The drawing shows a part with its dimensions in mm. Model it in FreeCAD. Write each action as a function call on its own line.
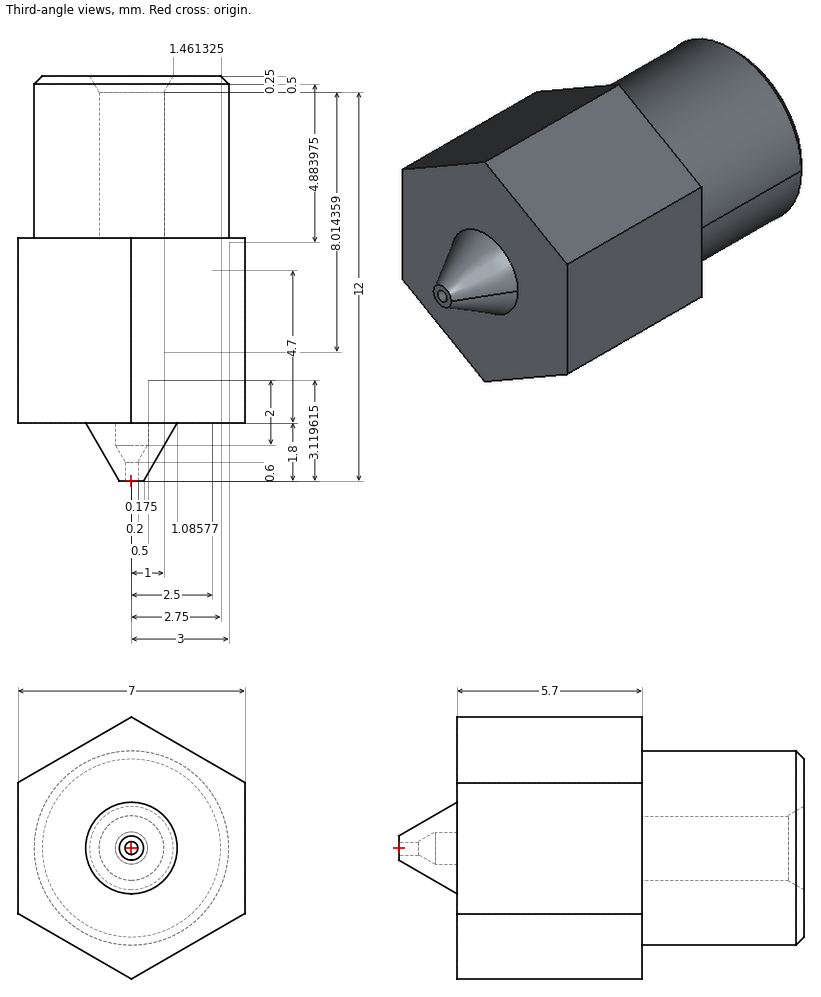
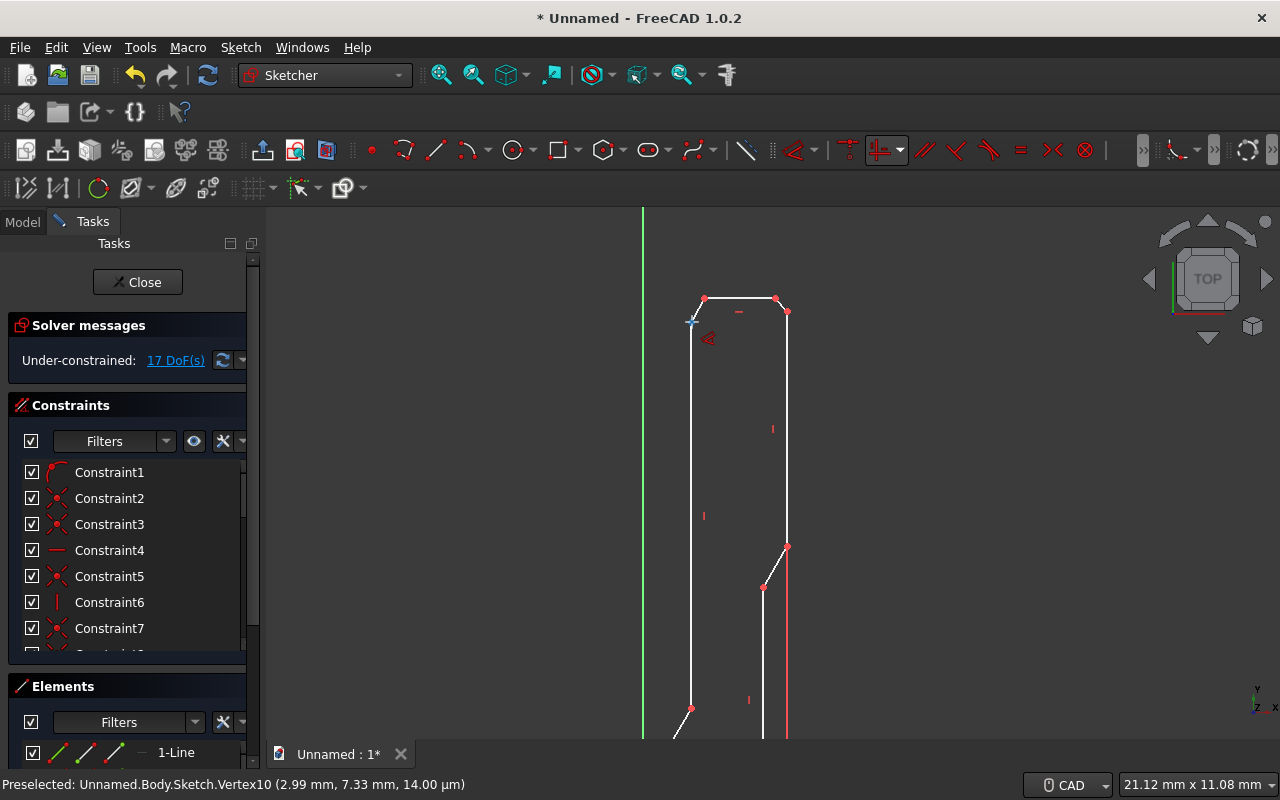
click(691, 322)
click(667, 288)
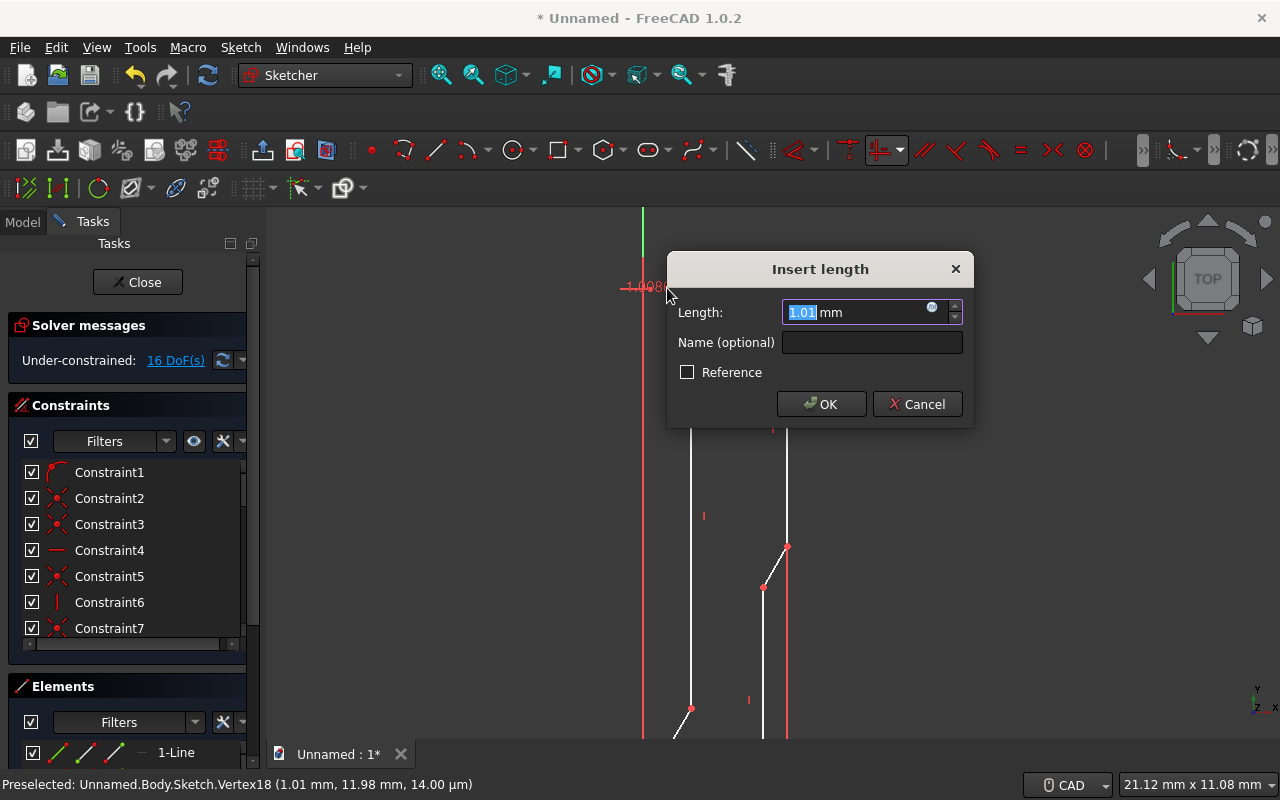
text(1)
key(Return)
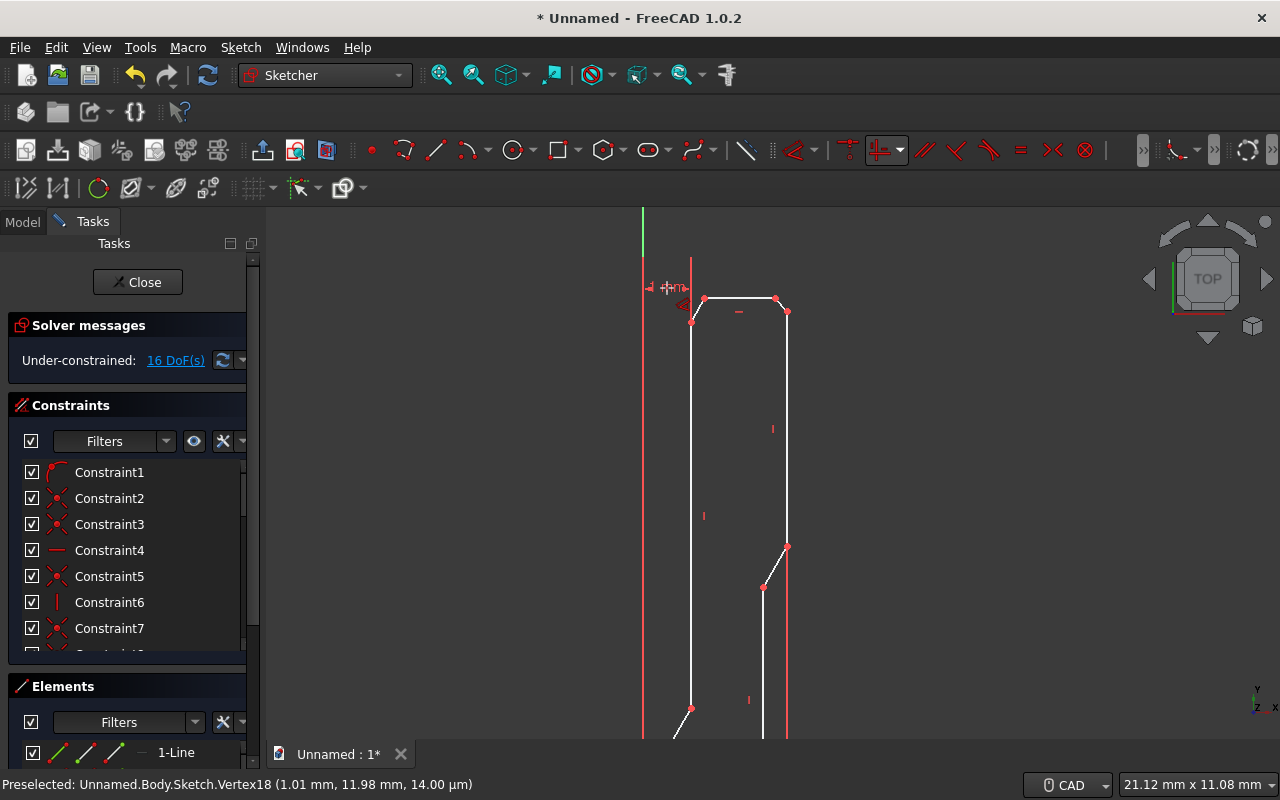
click(763, 655)
click(797, 649)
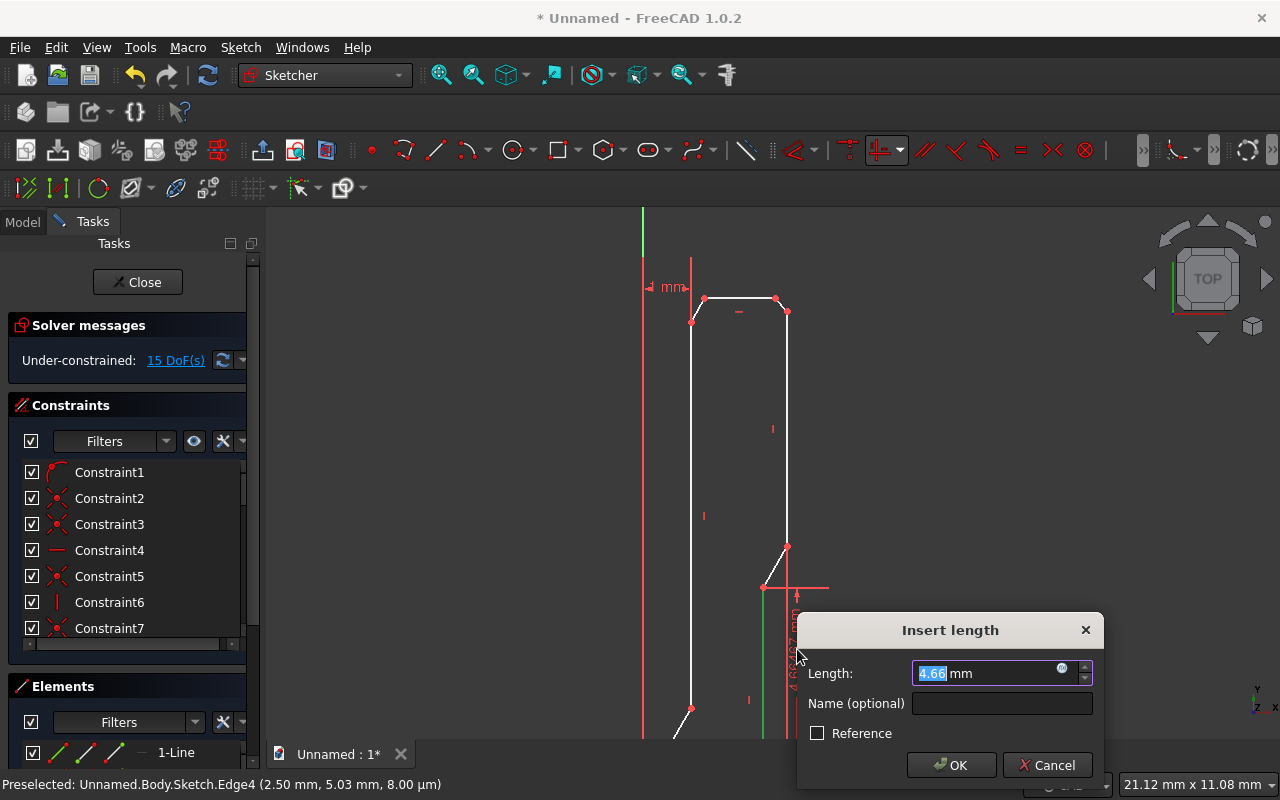
text(4.7)
key(Return)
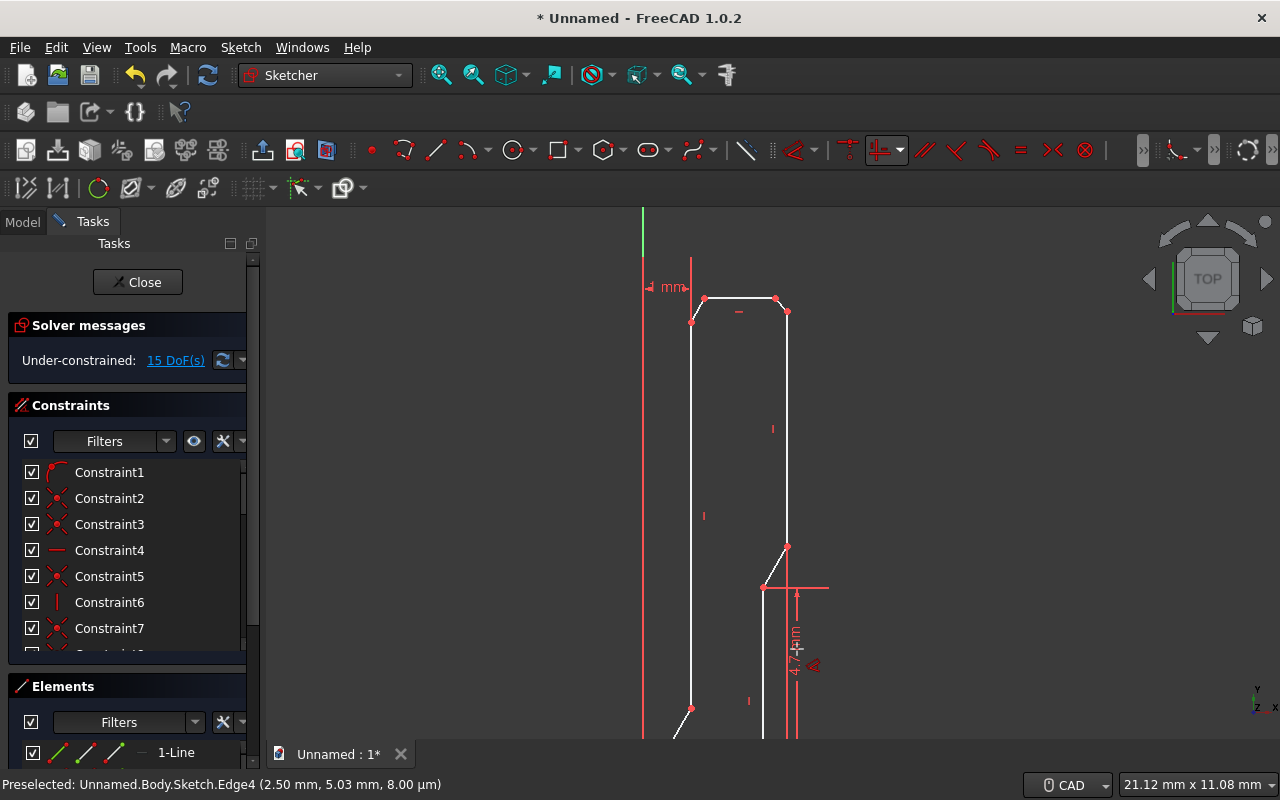
scroll(692, 321, down, 3)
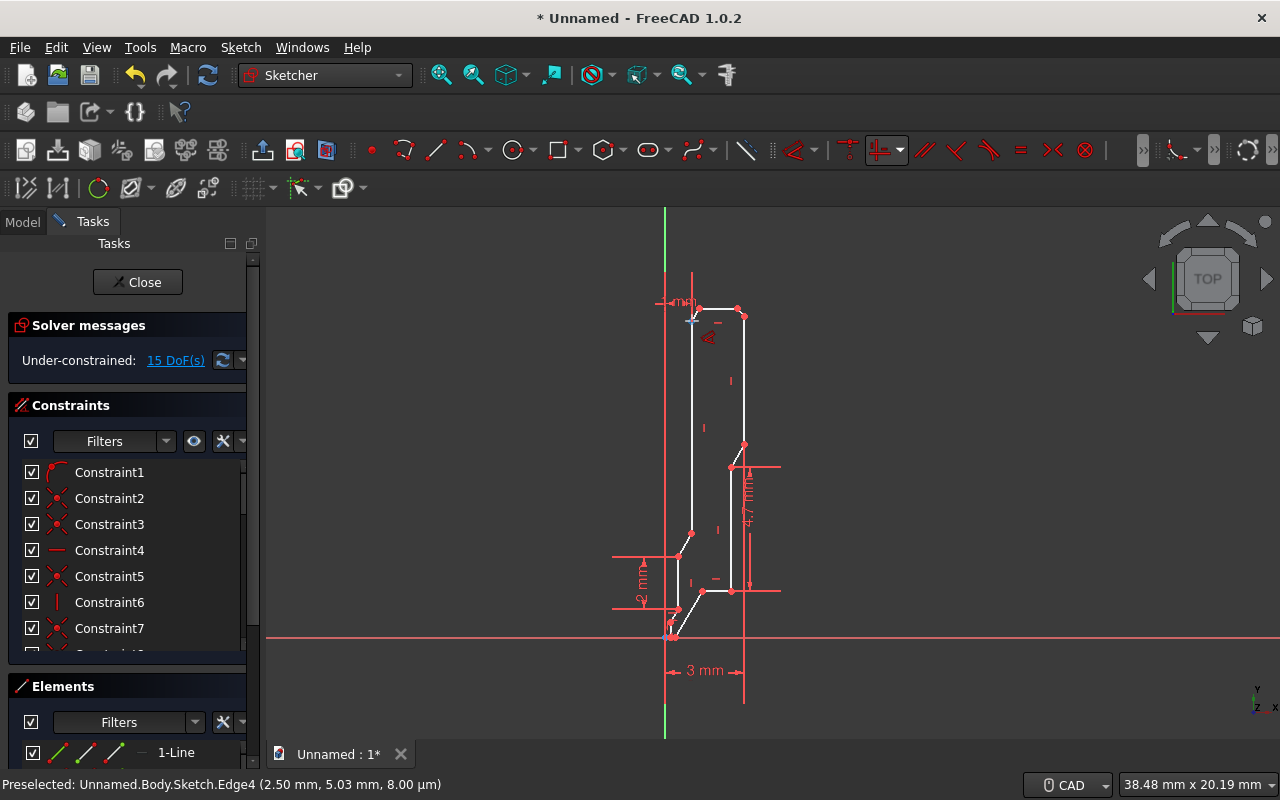
scroll(671, 628, up, 5)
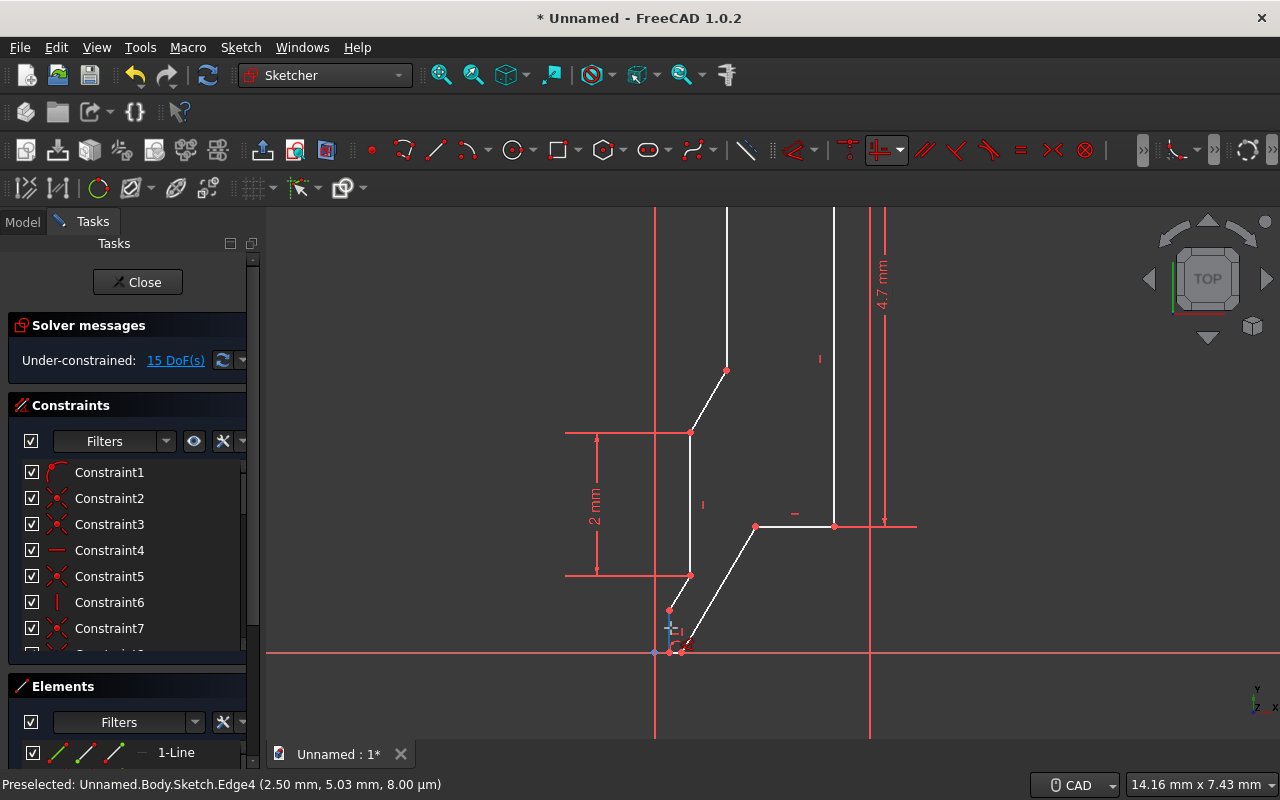
click(669, 627)
click(635, 632)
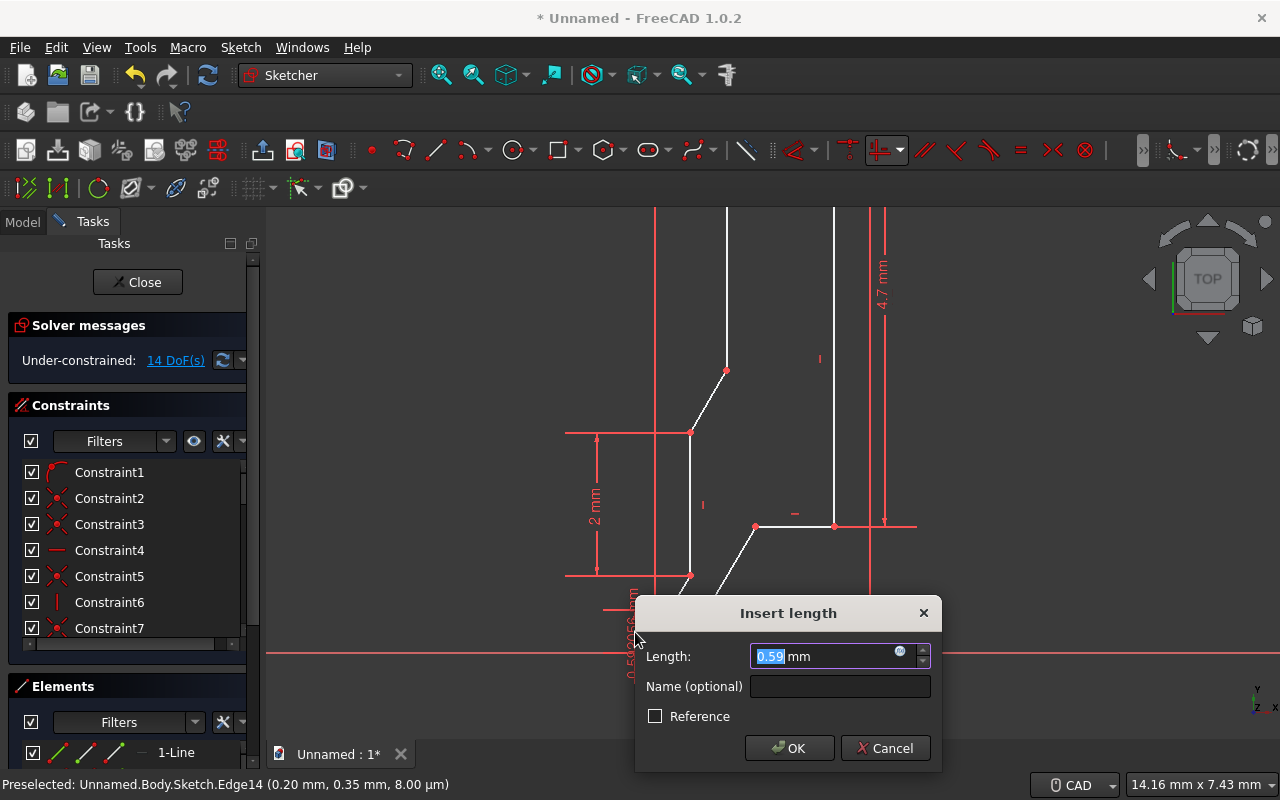
text(0.6)
key(Return)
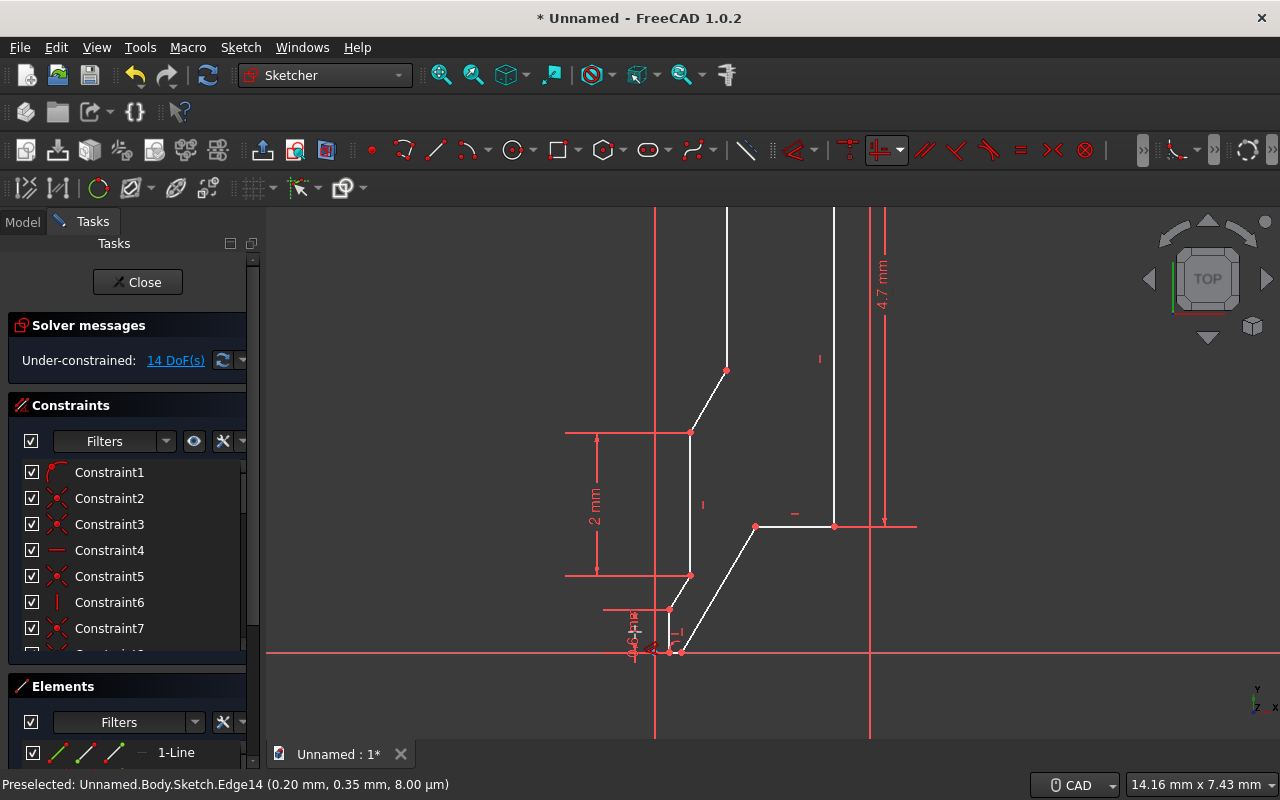
scroll(671, 629, down, 5)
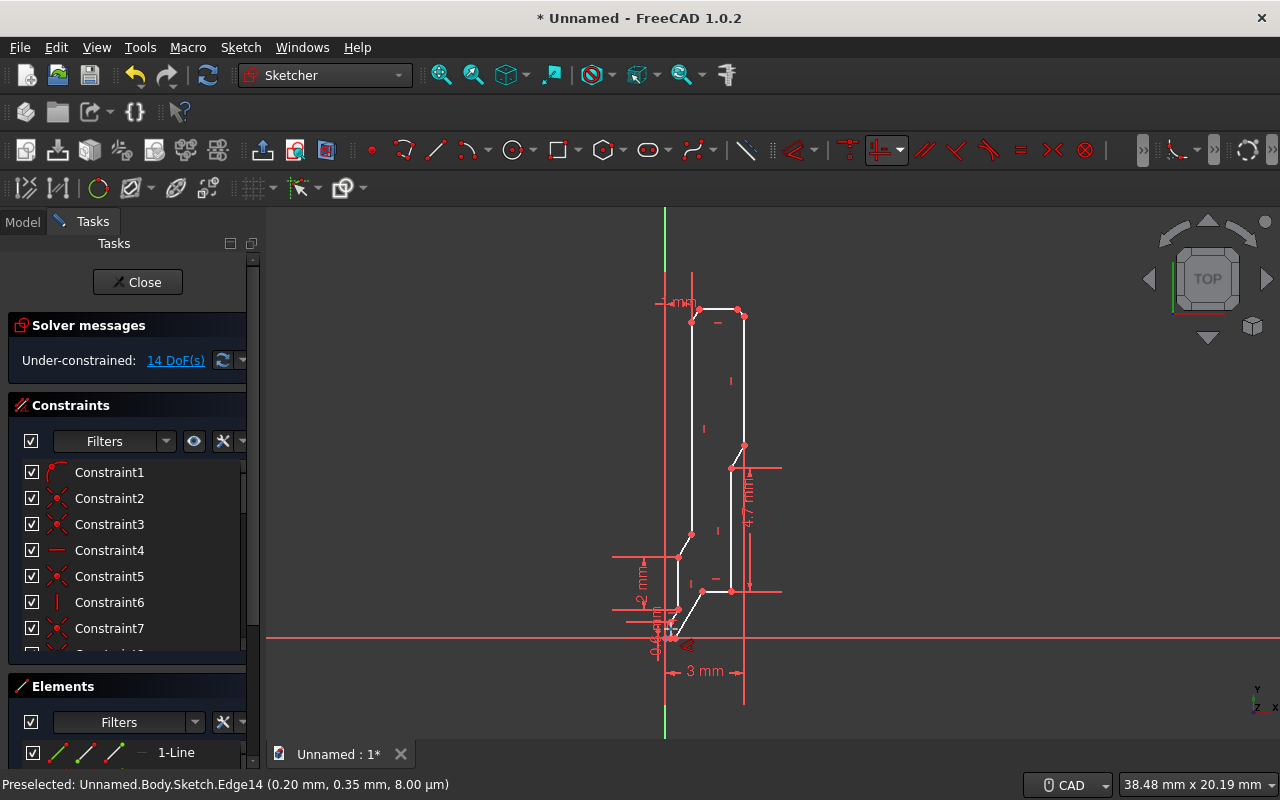
click(692, 322)
click(631, 480)